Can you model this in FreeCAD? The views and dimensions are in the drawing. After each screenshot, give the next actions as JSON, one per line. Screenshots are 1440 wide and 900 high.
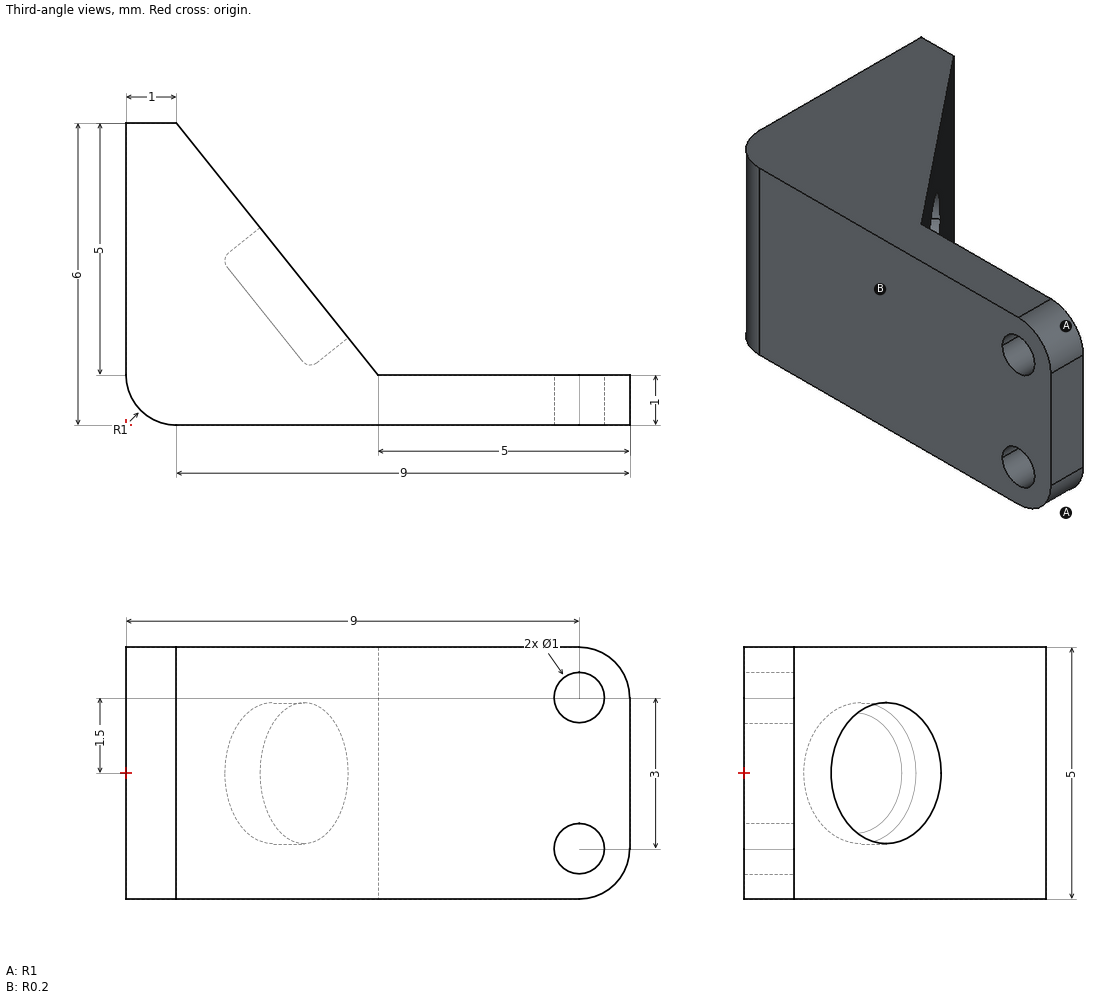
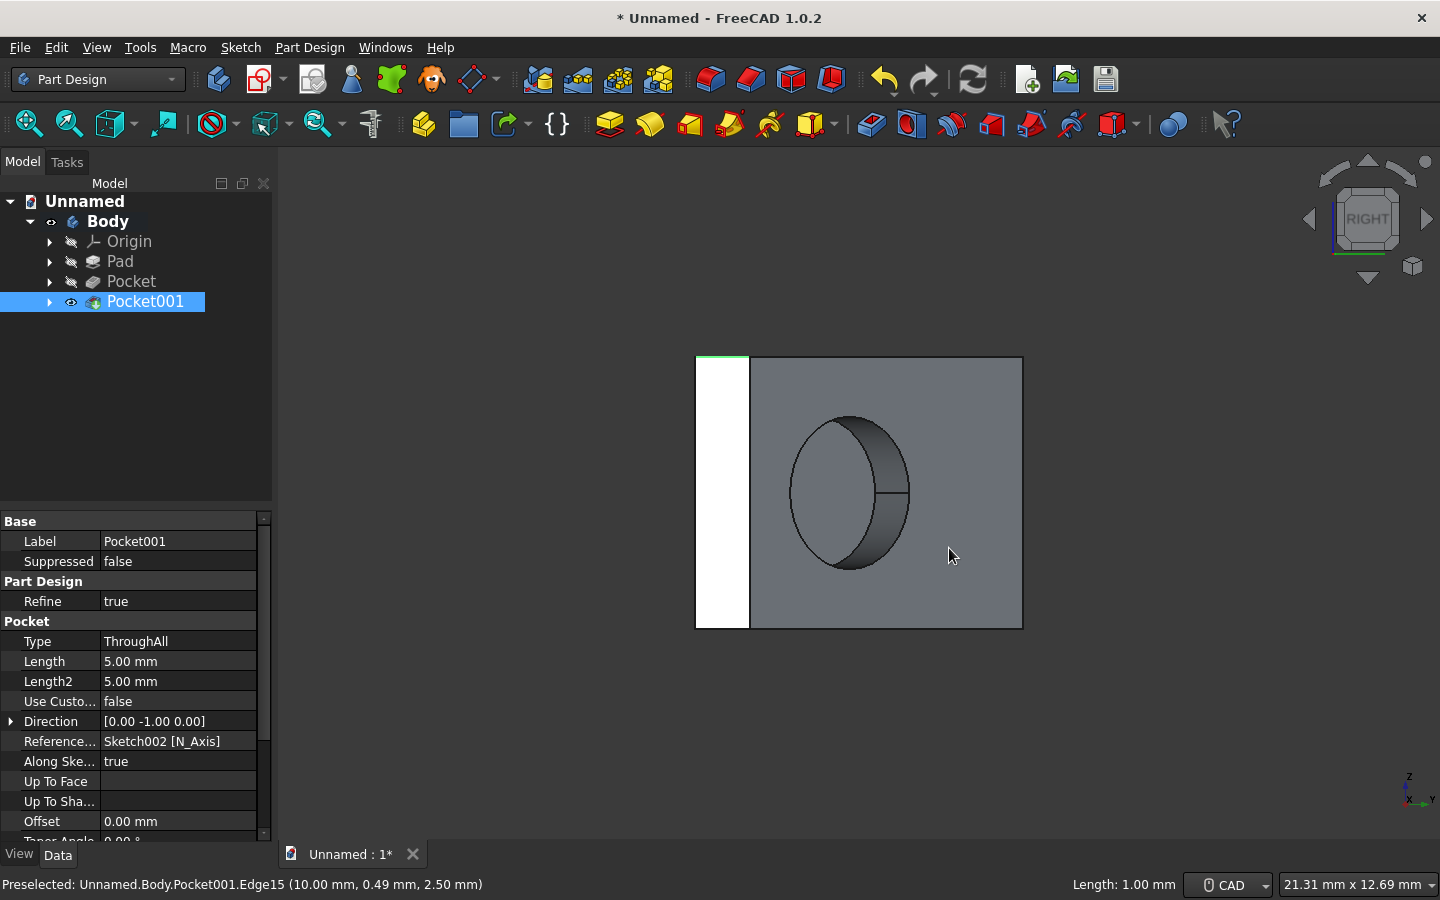
{"action": "left_click", "coordinate": [30, 124]}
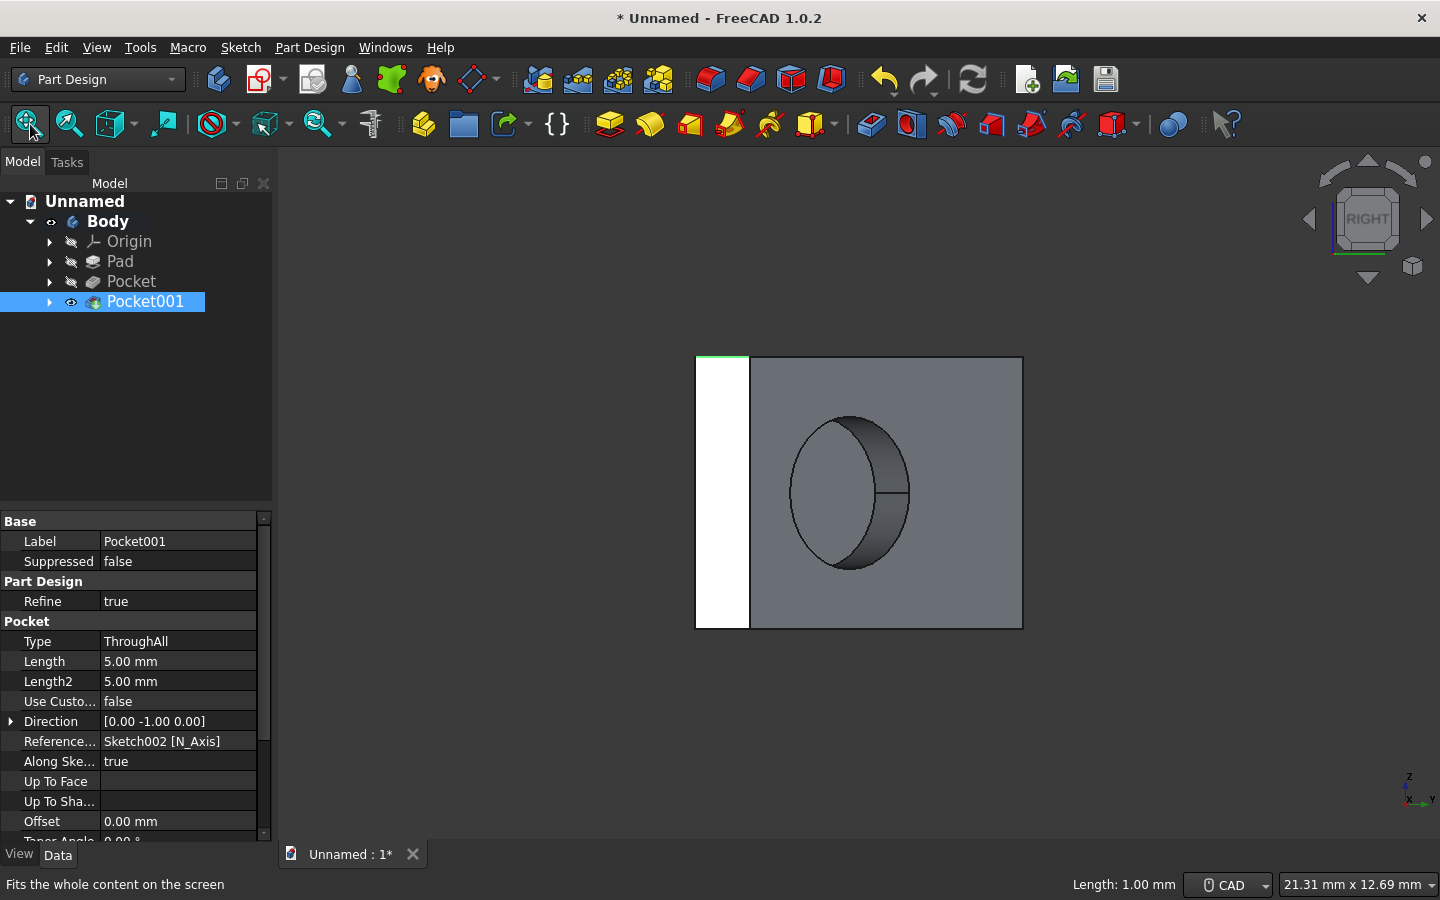
{"action": "left_click", "coordinate": [723, 628], "text": "ctrl"}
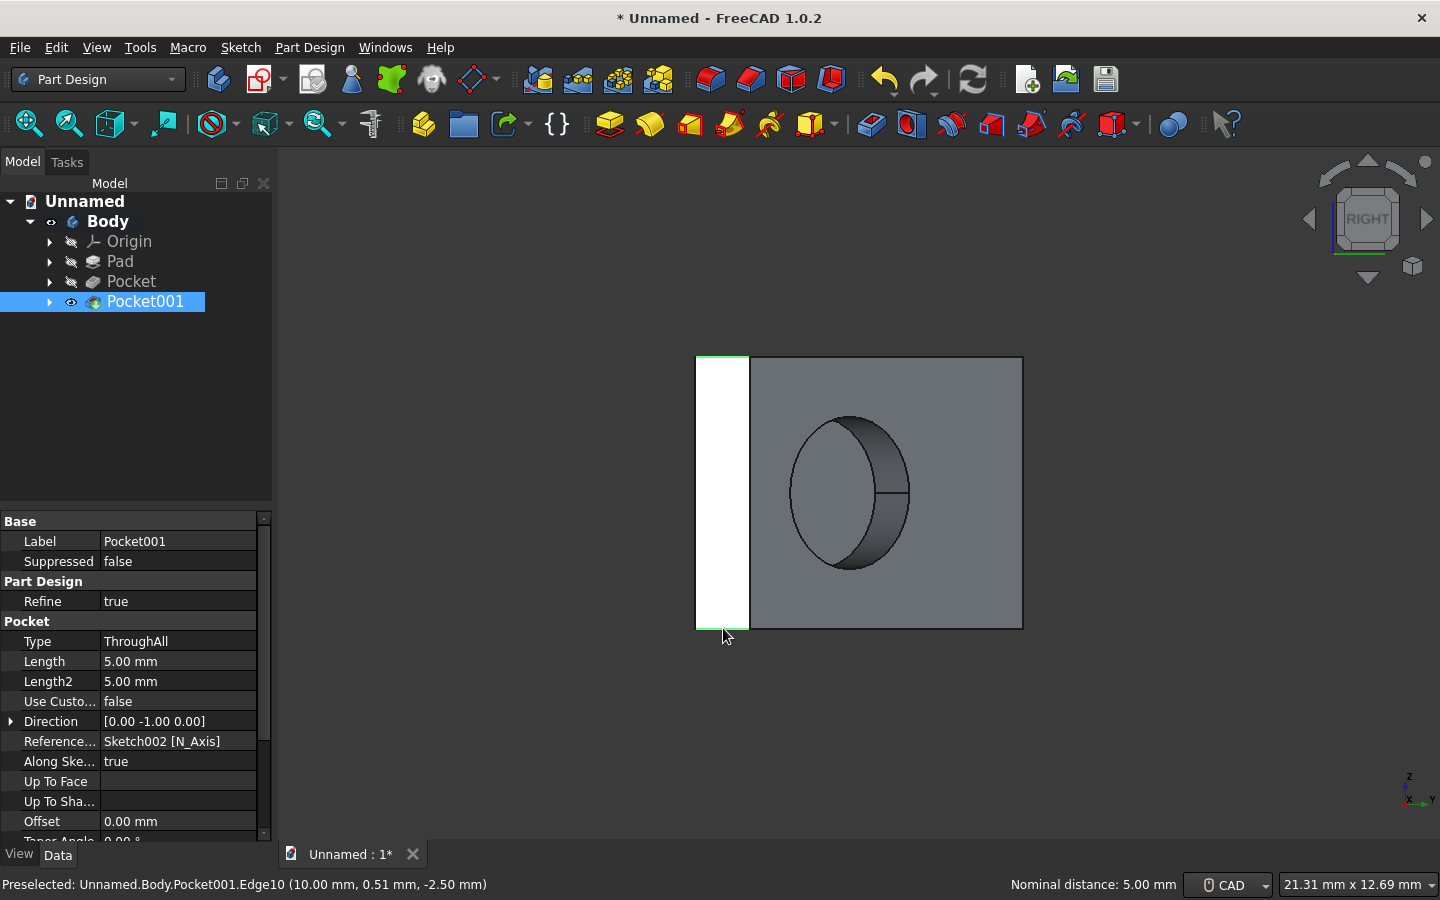
{"action": "left_click", "coordinate": [712, 80]}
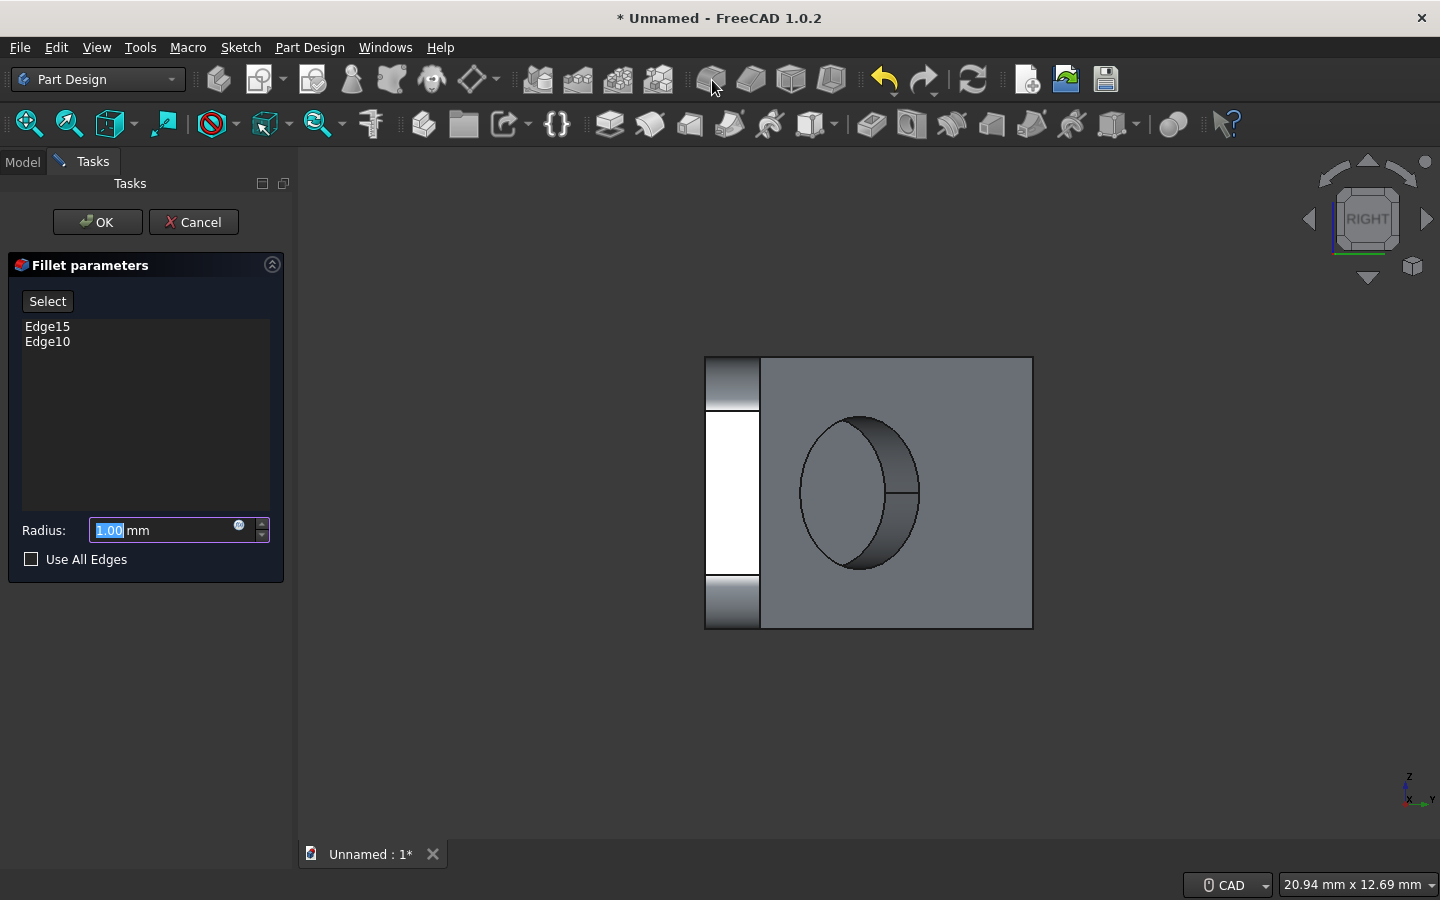
{"action": "type", "text": "1"}
{"action": "key", "text": "Tab"}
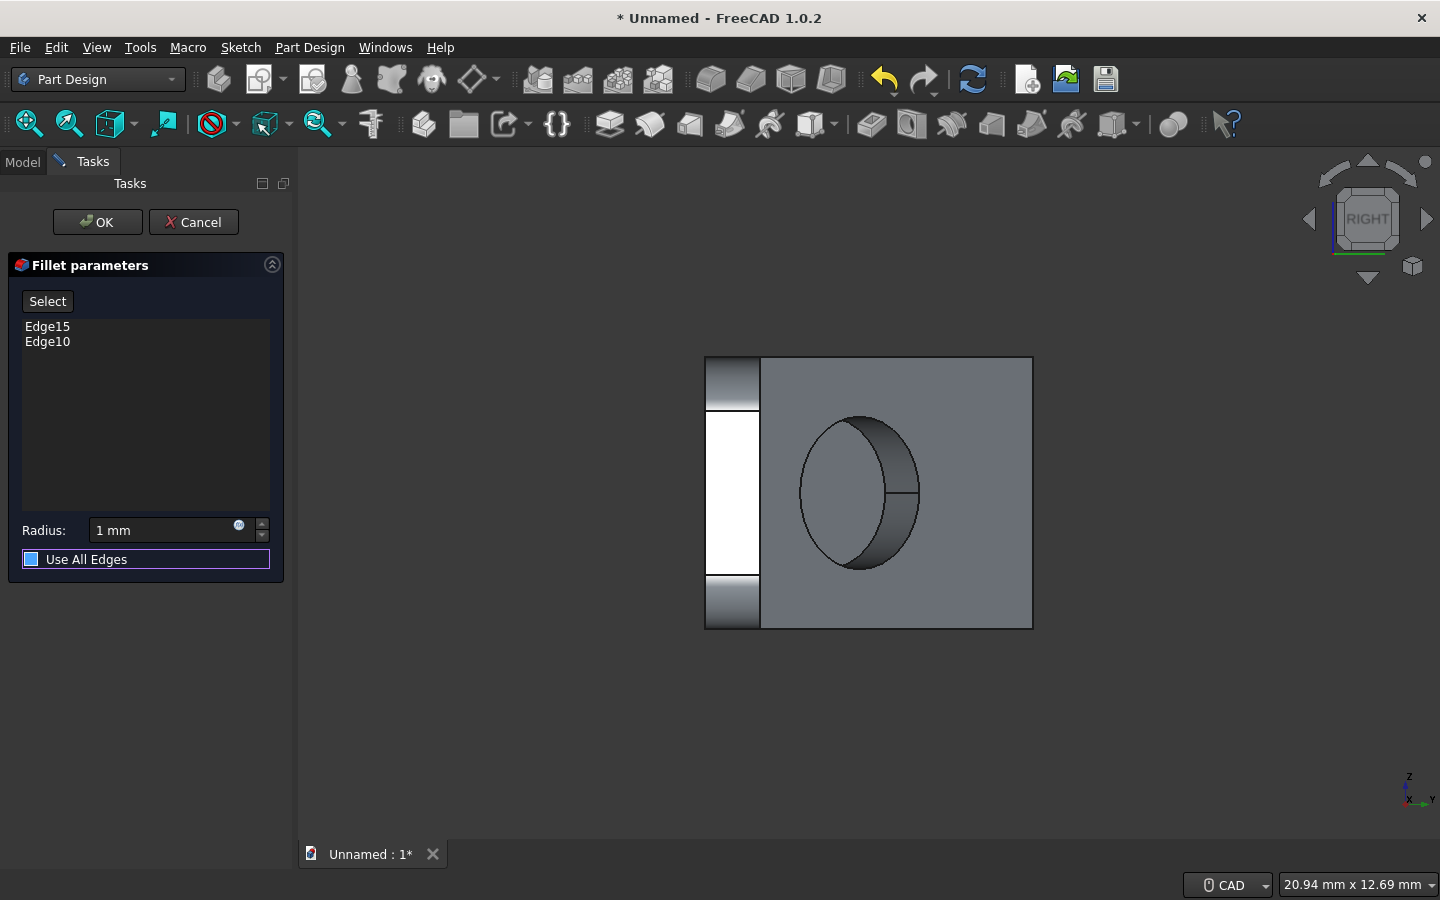
{"action": "left_click", "coordinate": [98, 222]}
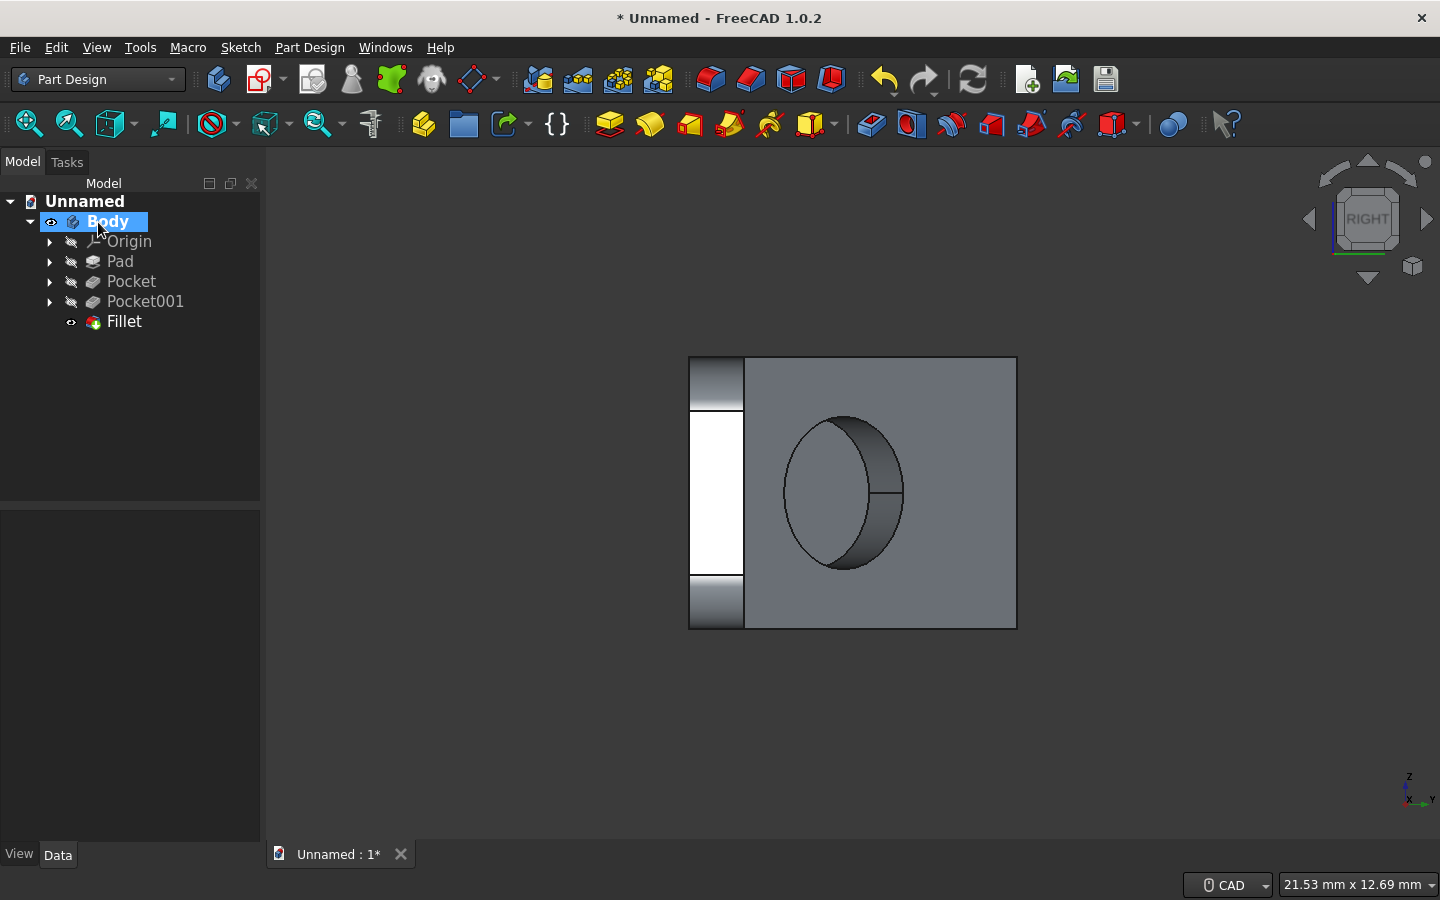
{"action": "left_click", "coordinate": [30, 124]}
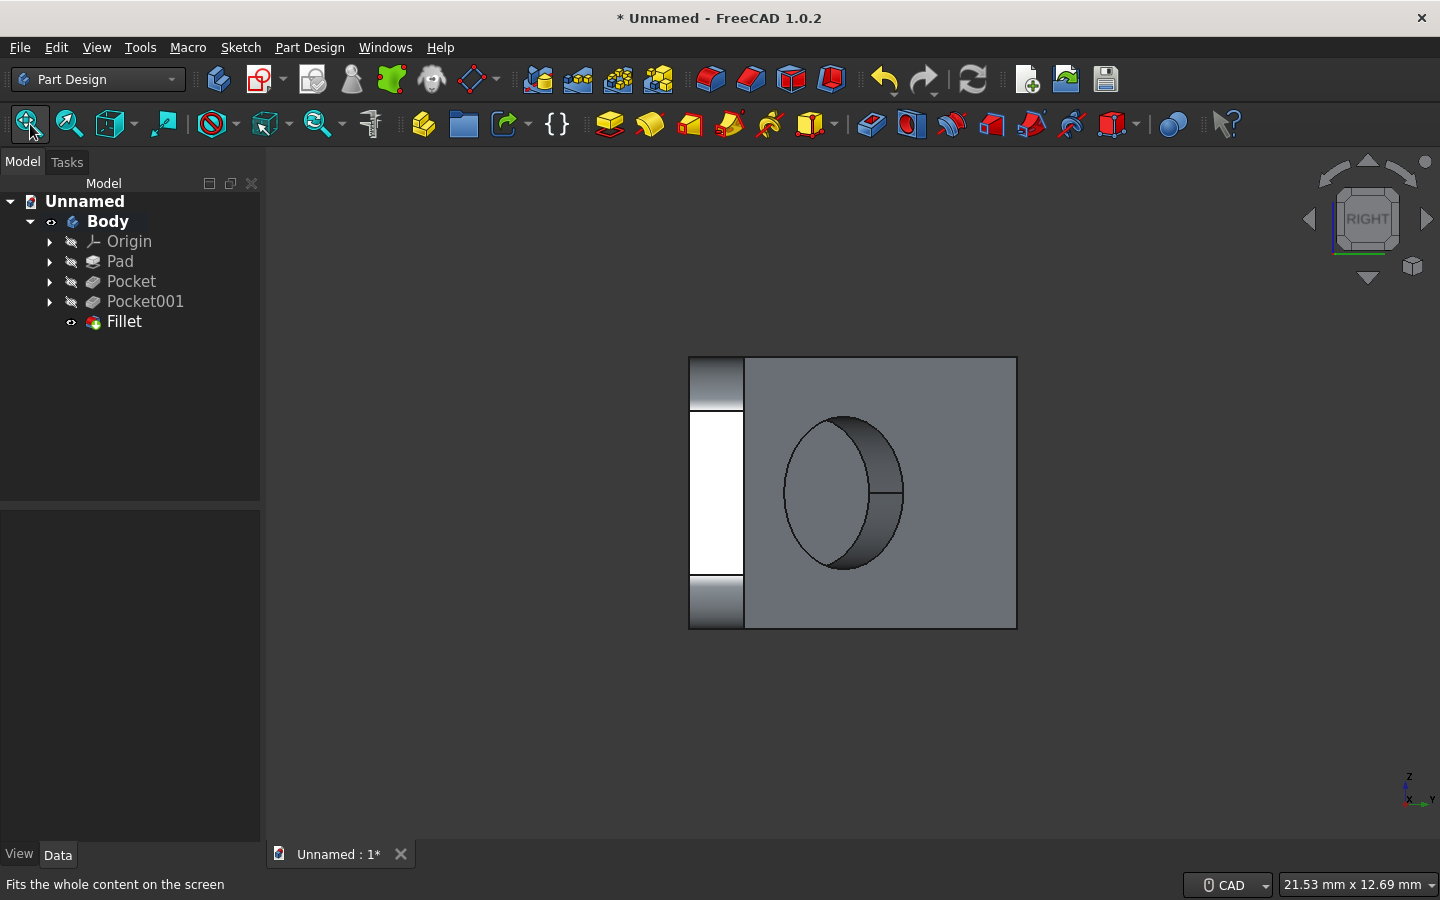
{"action": "key", "text": "0"}